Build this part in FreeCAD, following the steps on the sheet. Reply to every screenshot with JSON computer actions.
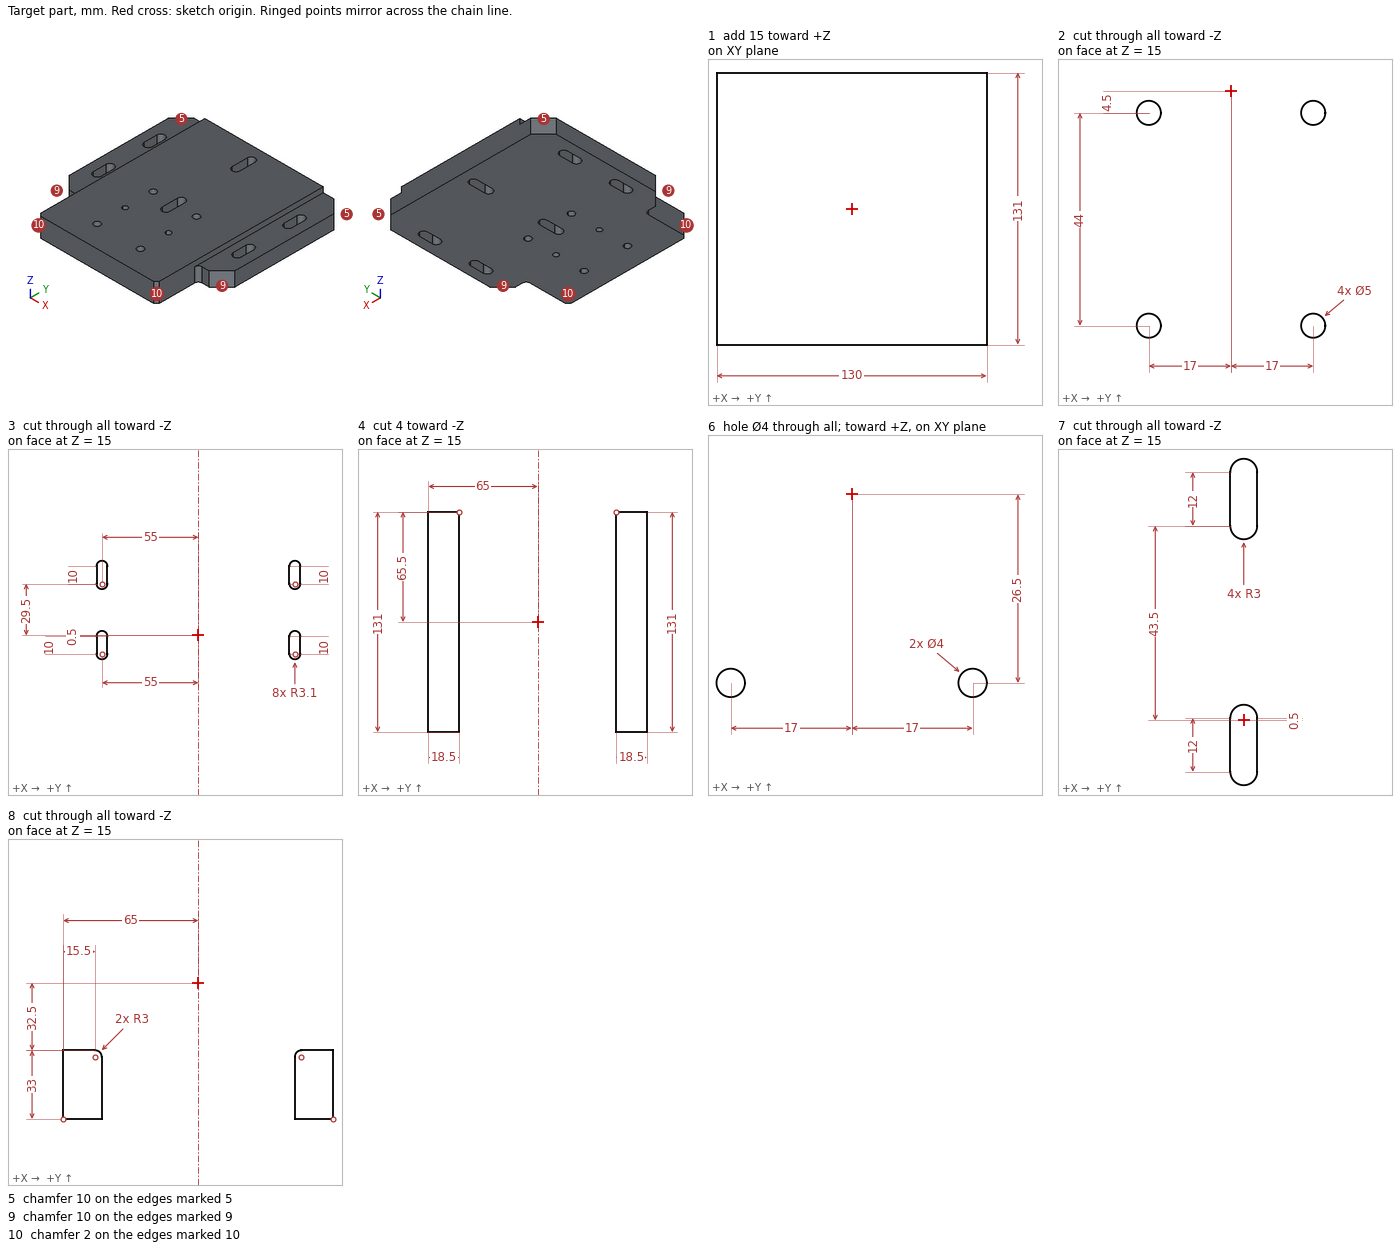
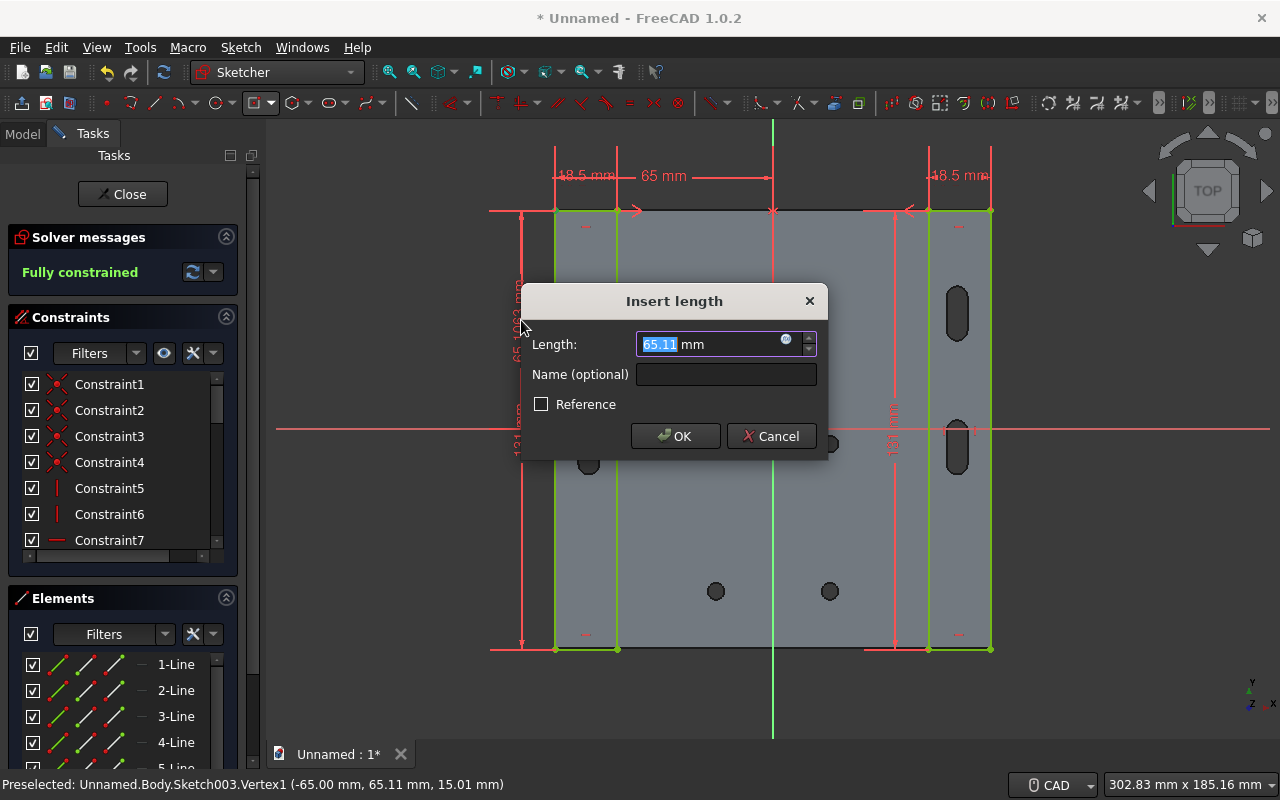
{"action": "type", "text": "65.5"}
{"action": "key", "text": "Return"}
{"action": "key", "text": "Escape"}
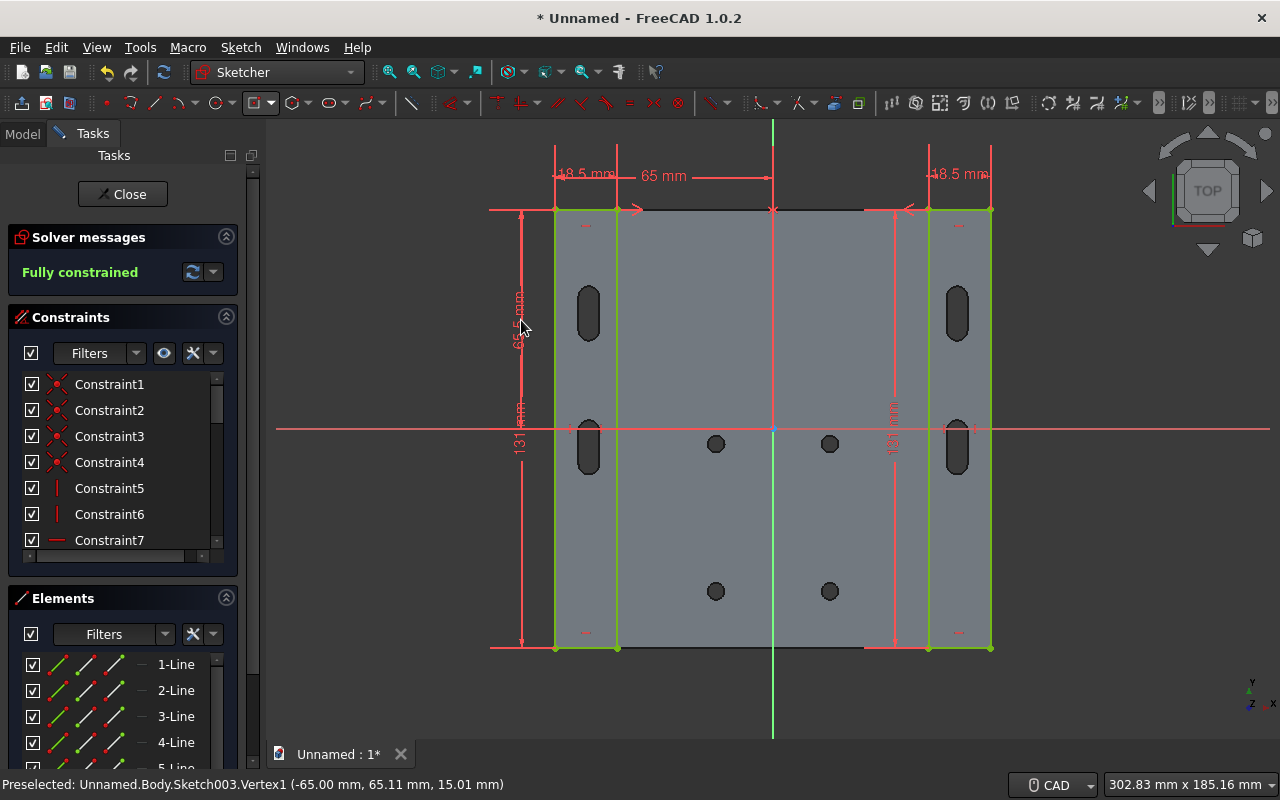
{"action": "left_click", "coordinate": [123, 194]}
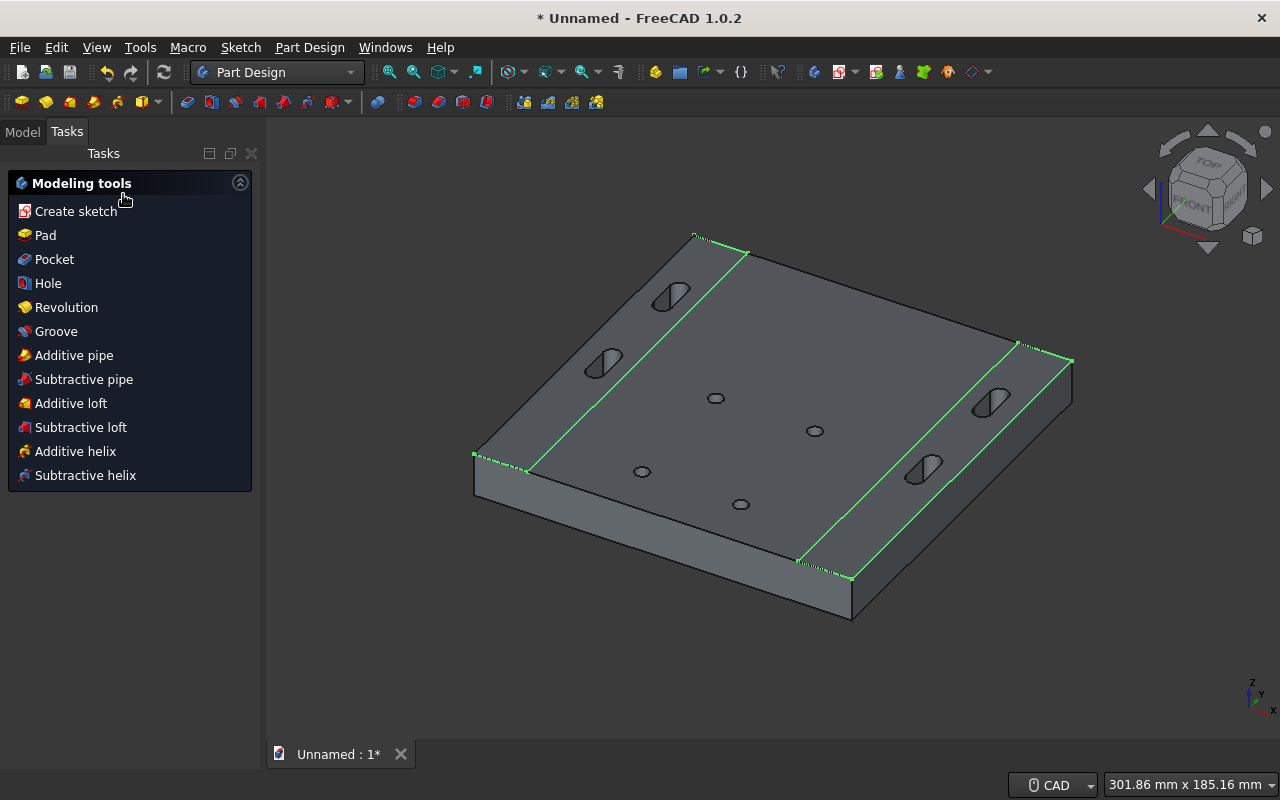
{"action": "left_click", "coordinate": [188, 102]}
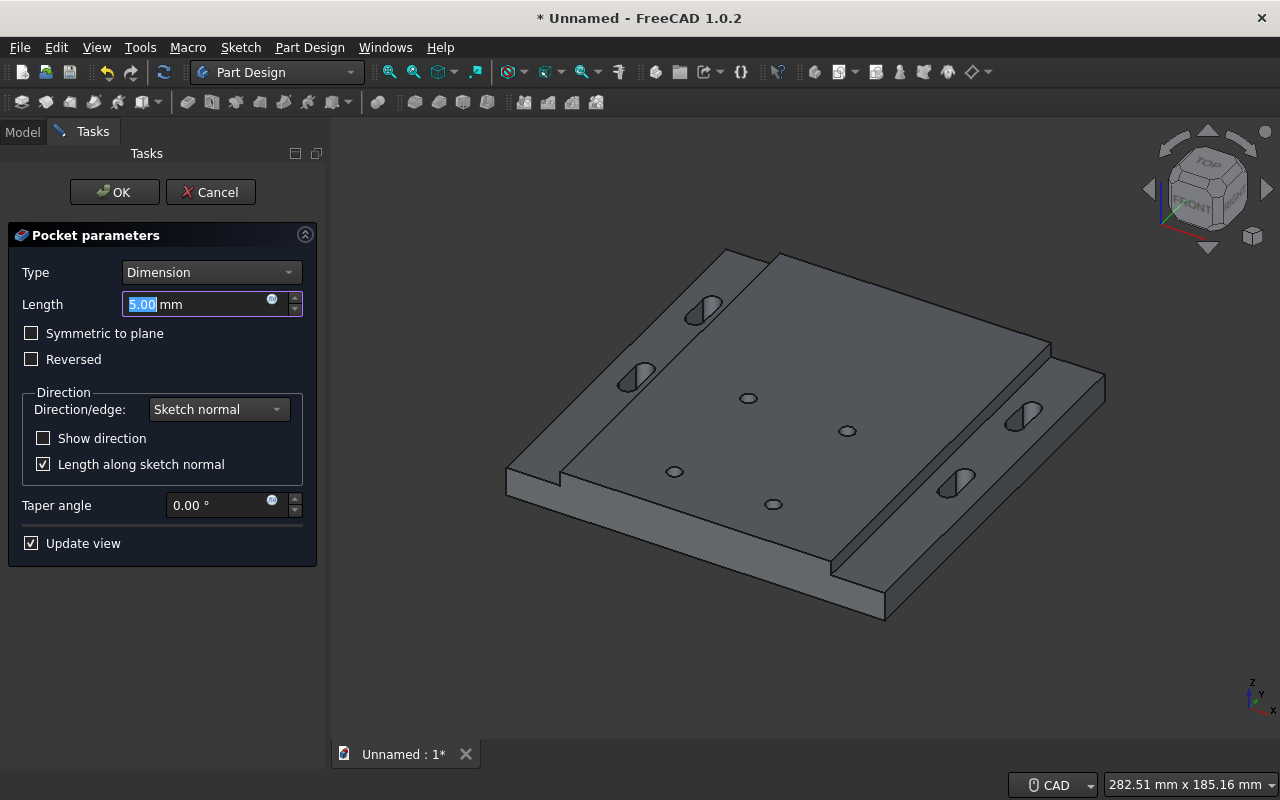
{"action": "type", "text": "4"}
{"action": "key", "text": "Tab"}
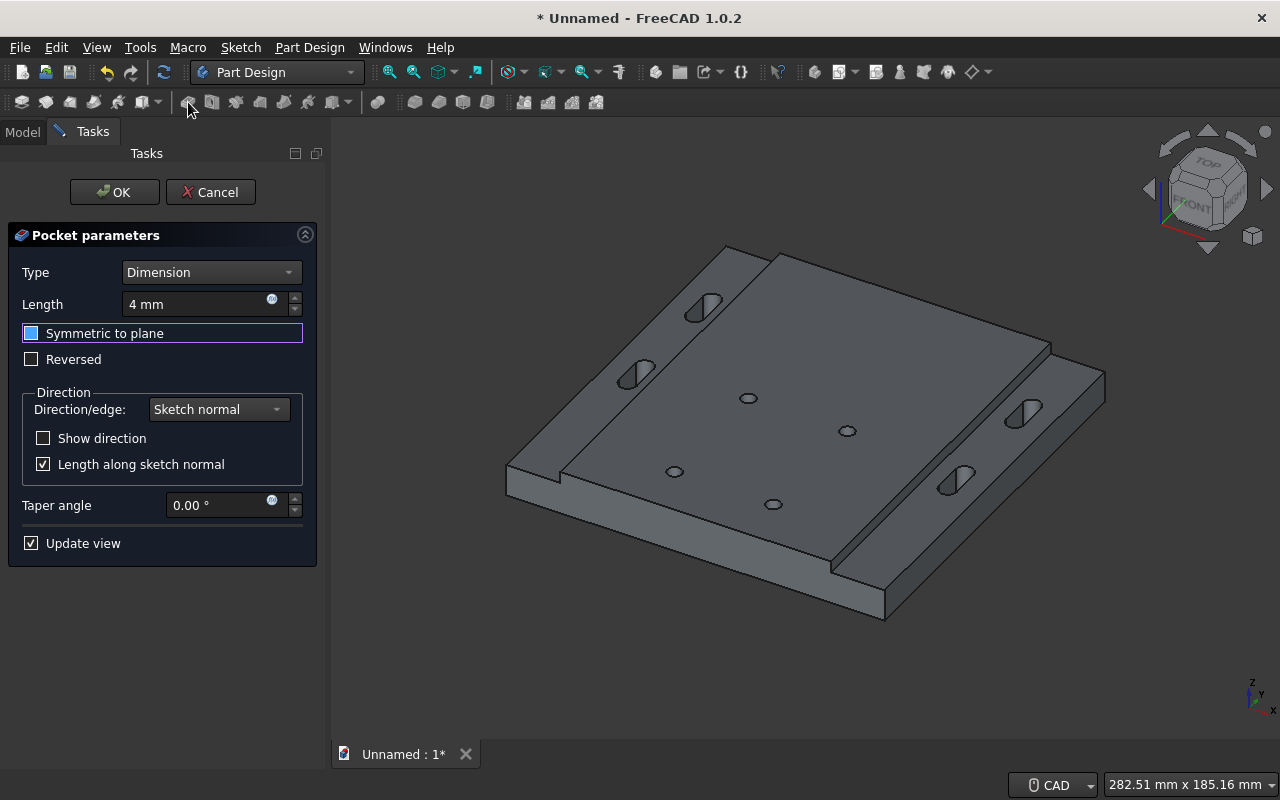
{"action": "left_click", "coordinate": [115, 192]}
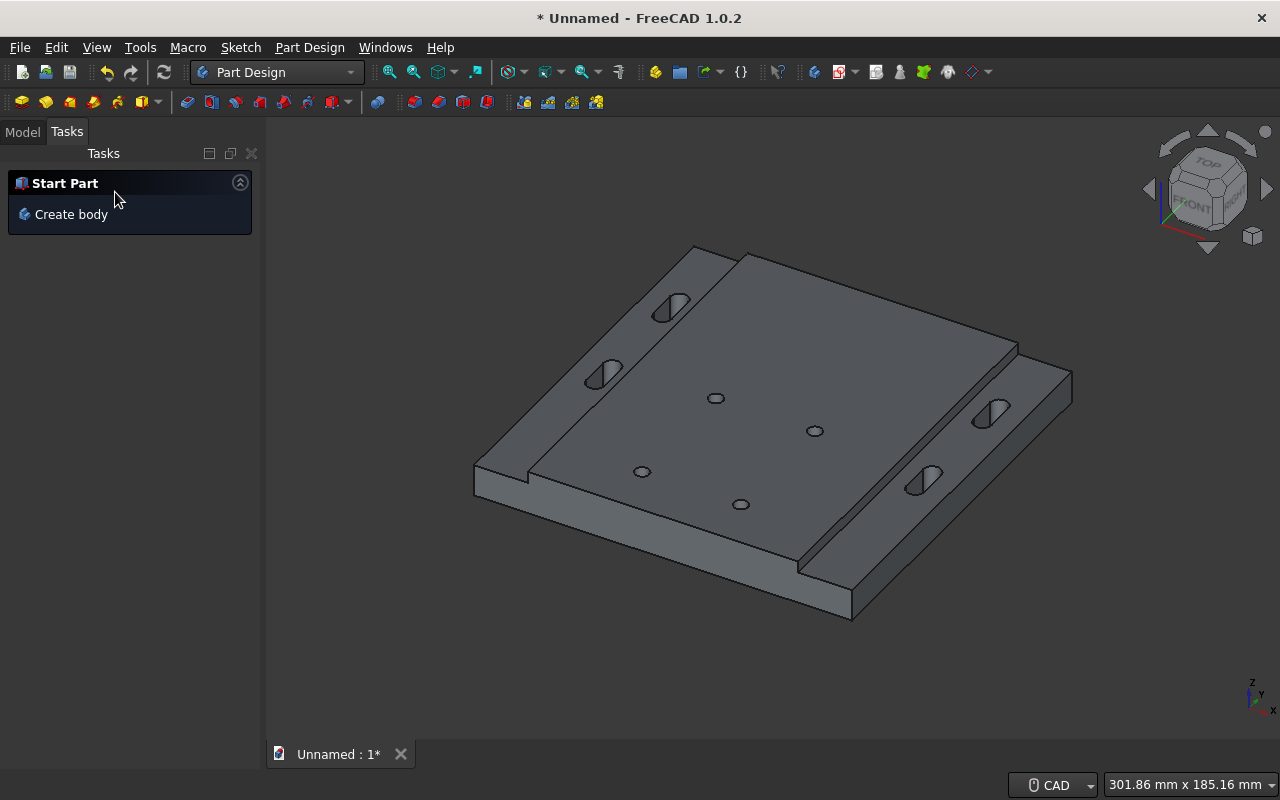
{"action": "key", "text": "0"}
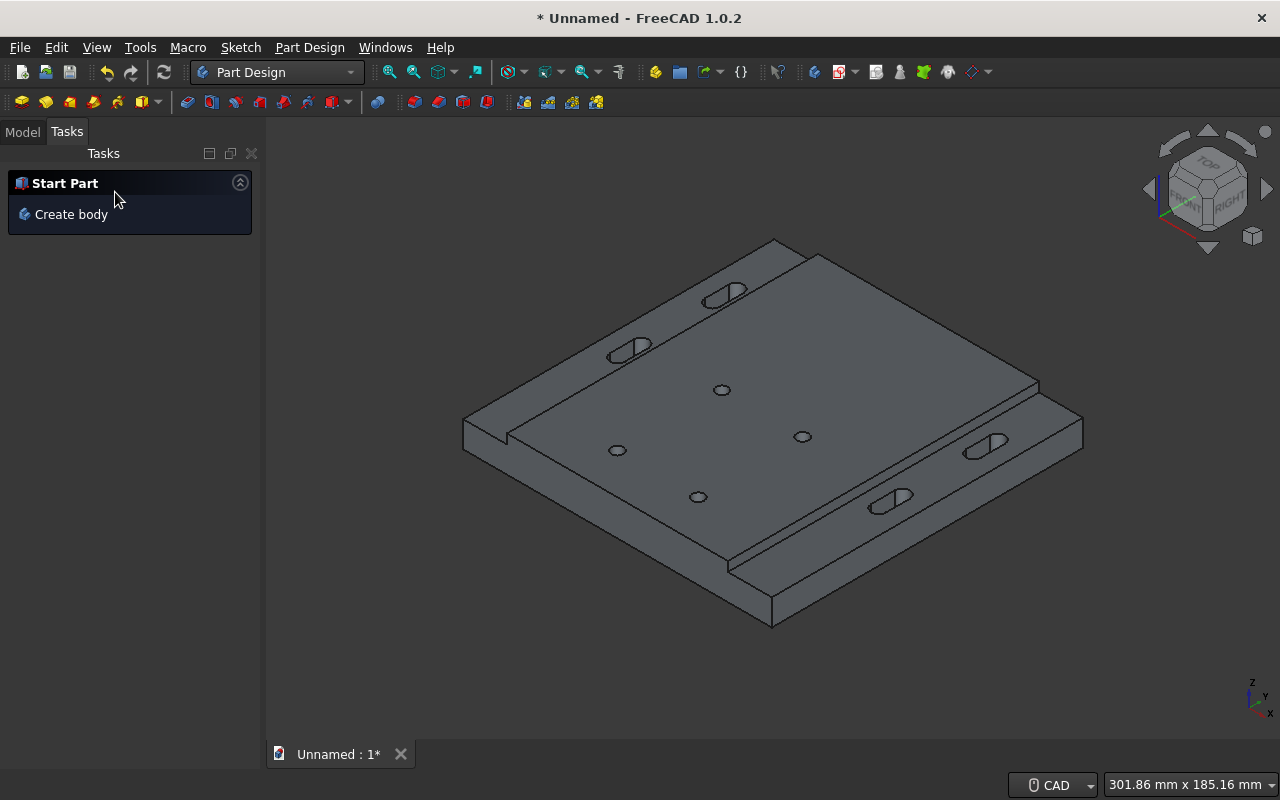
{"action": "key", "text": "2"}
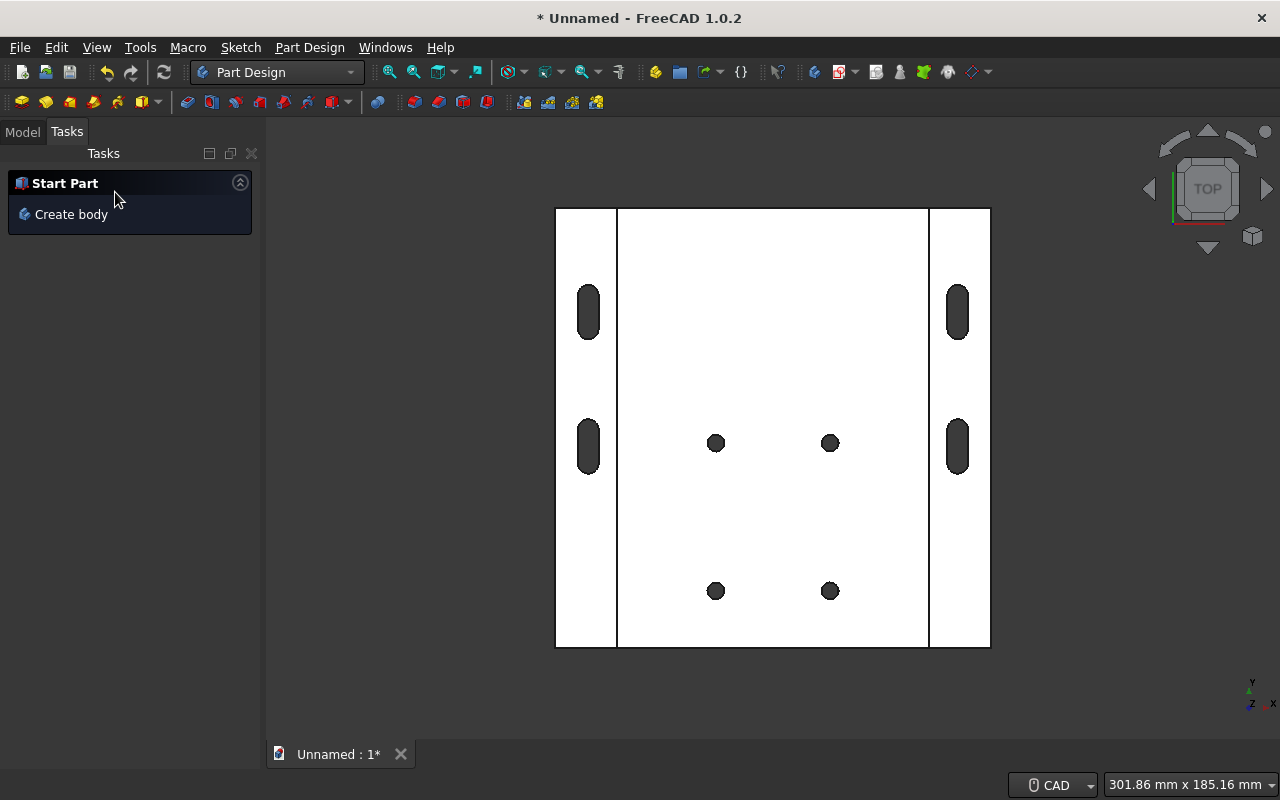
{"action": "key", "text": "1"}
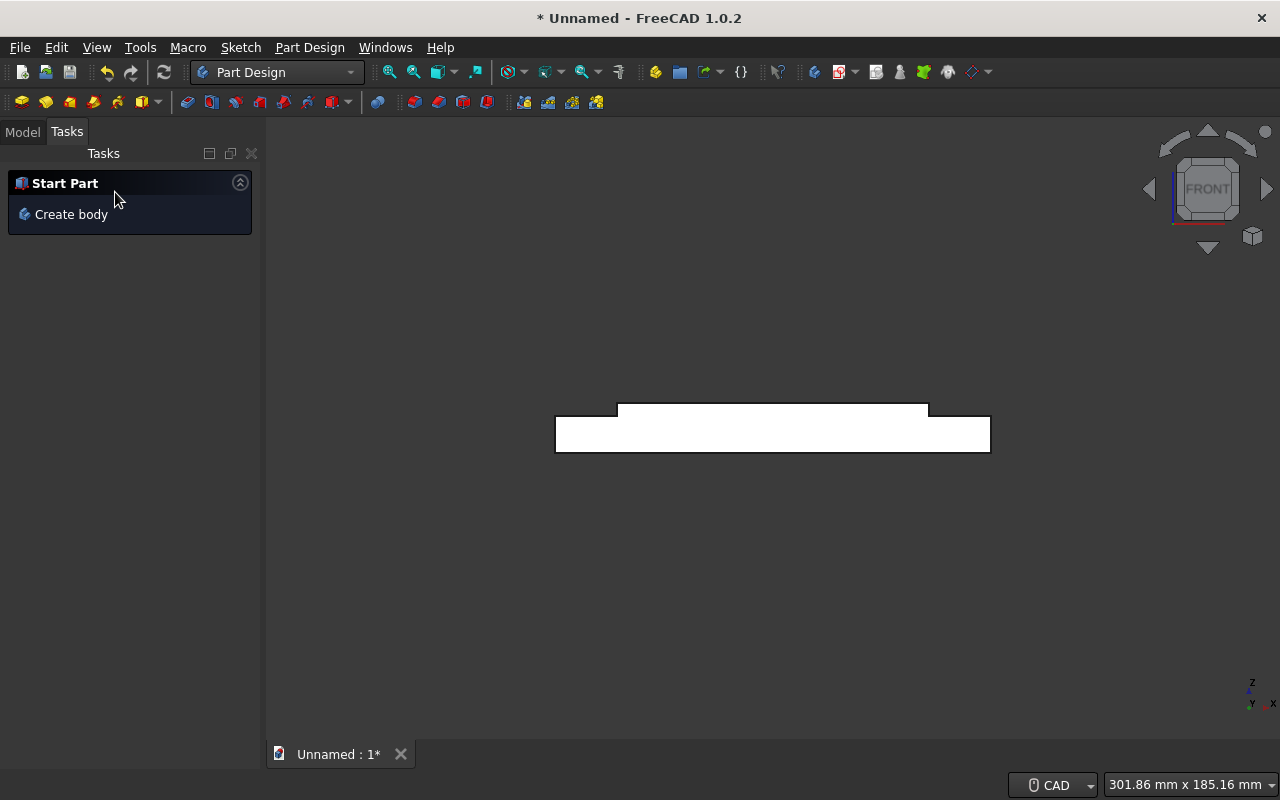
{"action": "key", "text": "v f"}